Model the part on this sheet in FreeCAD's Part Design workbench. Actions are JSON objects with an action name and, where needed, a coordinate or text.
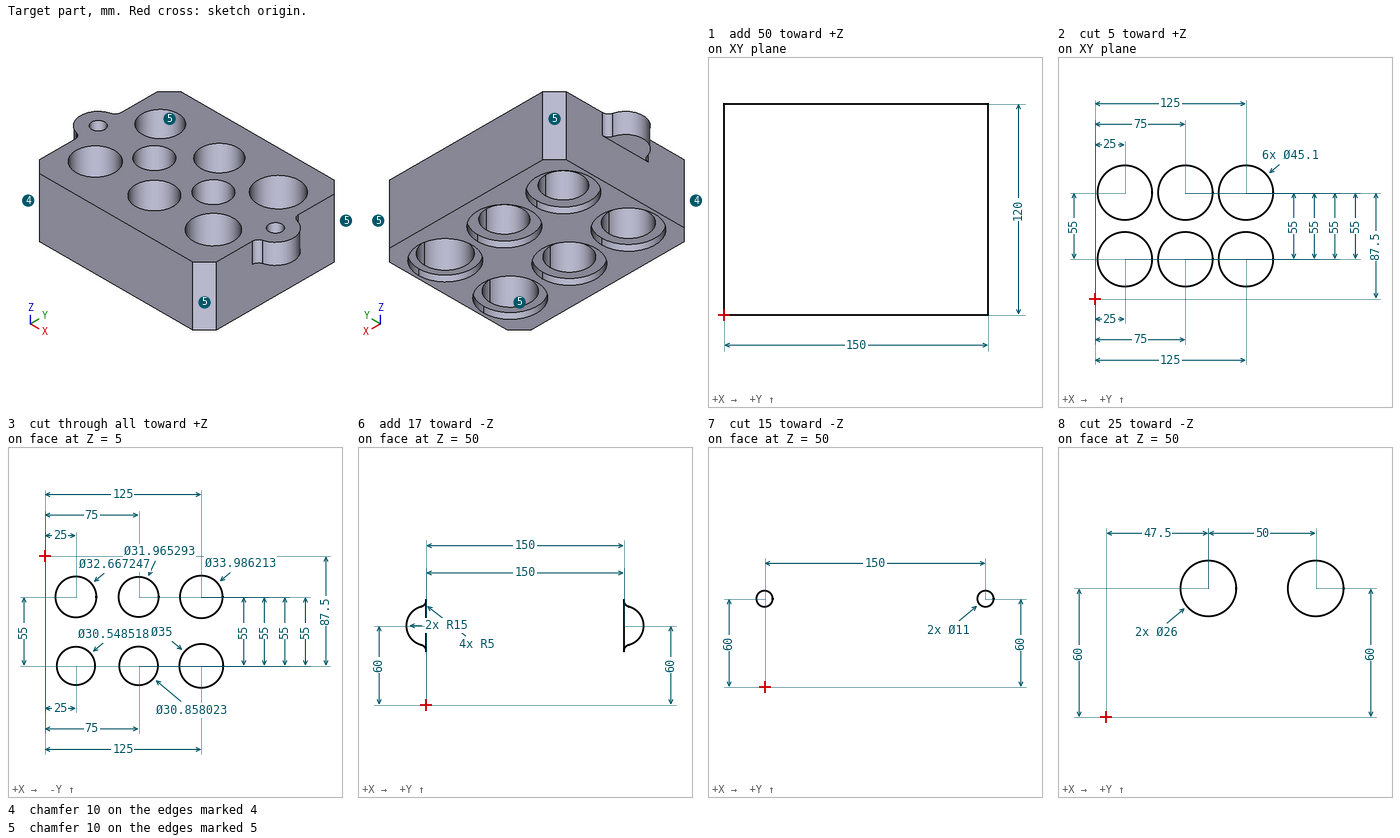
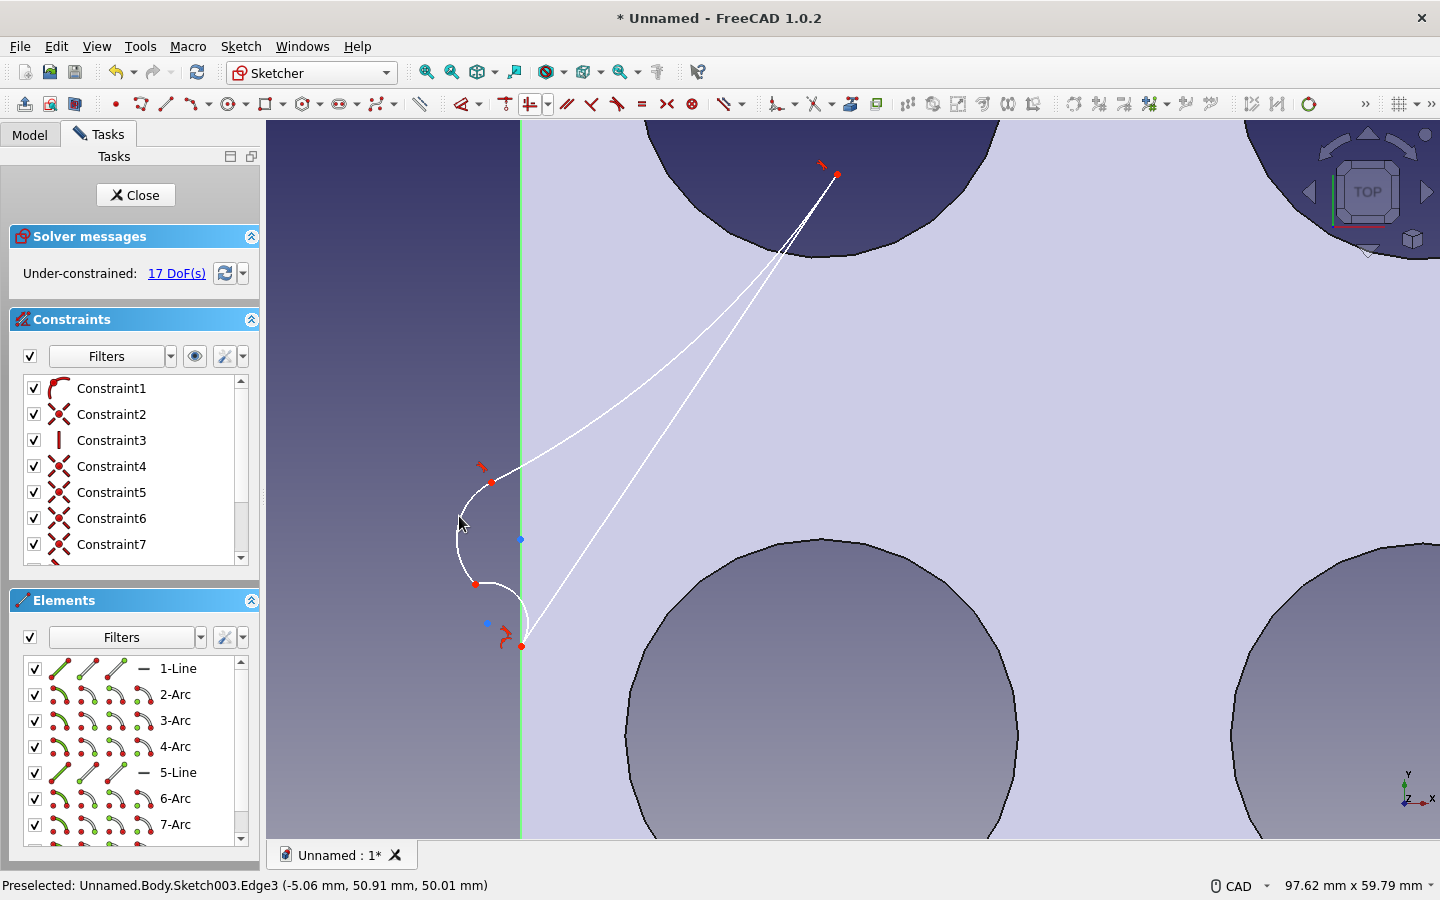
{"action": "left_click", "coordinate": [465, 507]}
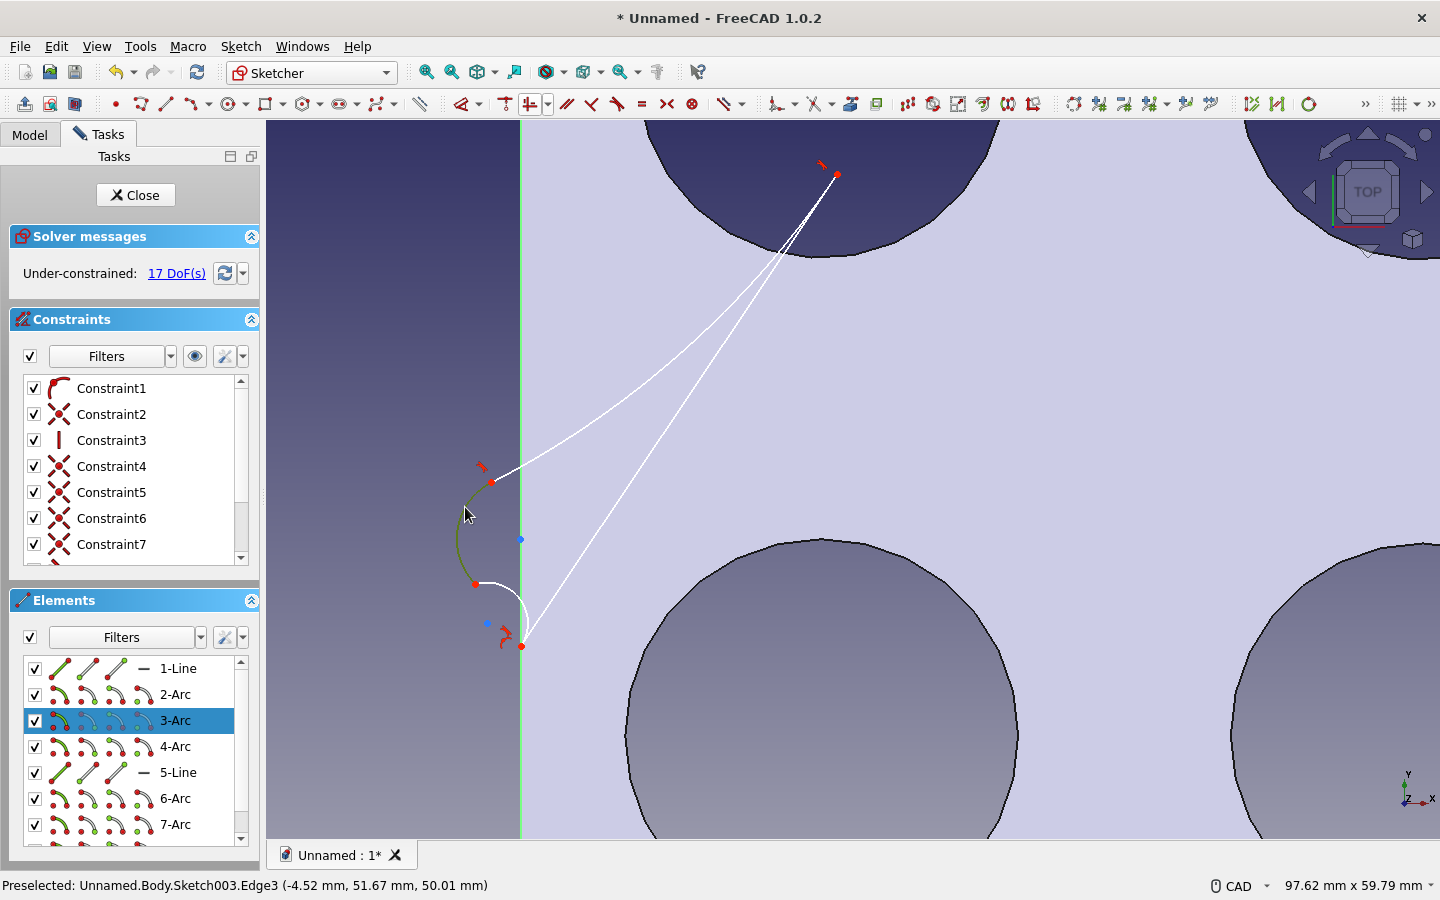
{"action": "left_click", "coordinate": [505, 587]}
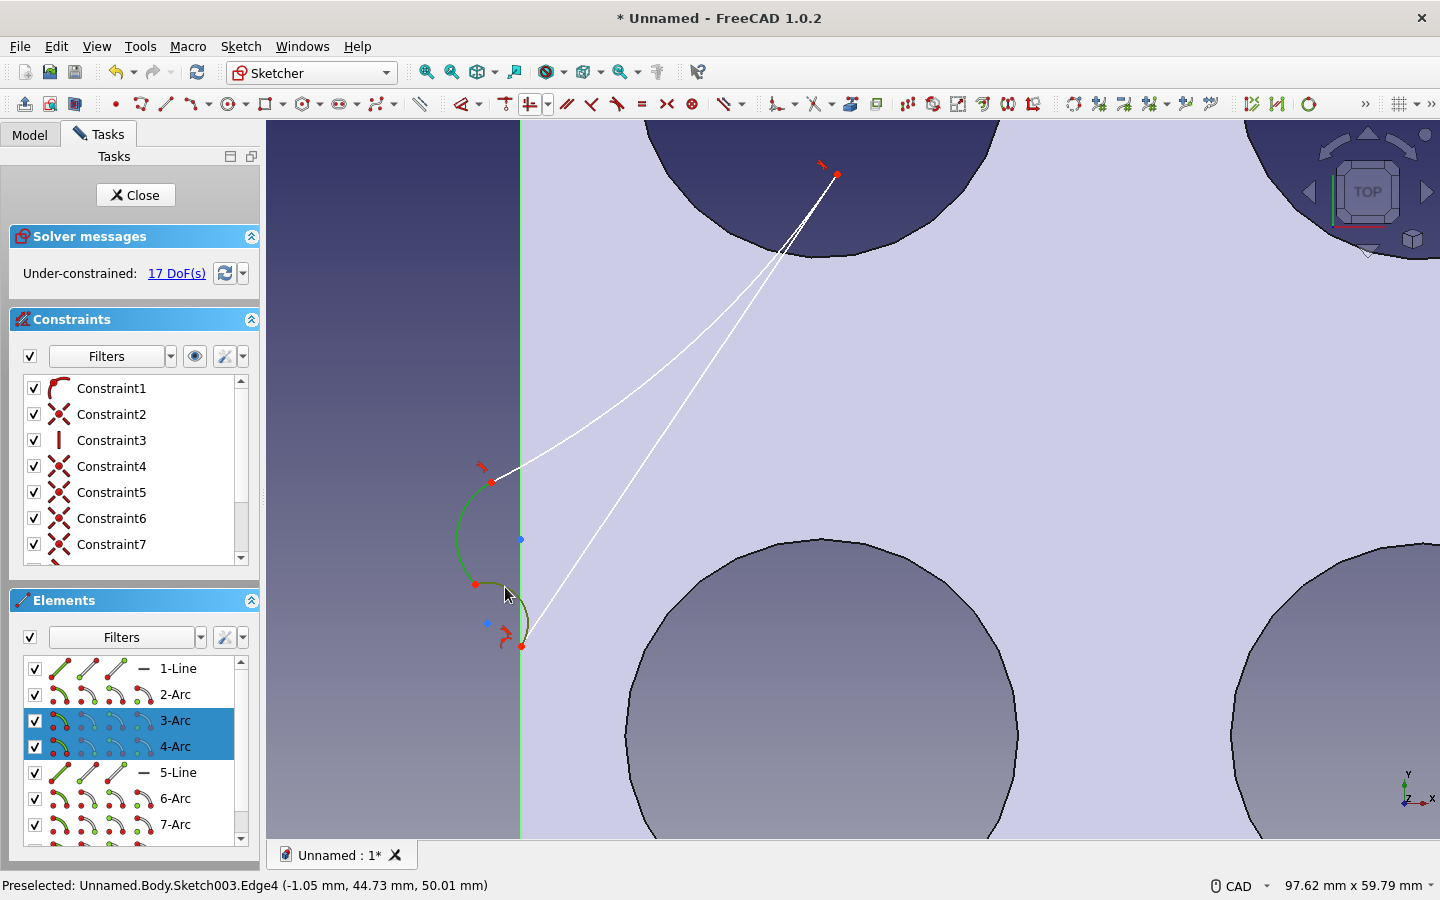
{"action": "left_click", "coordinate": [617, 104]}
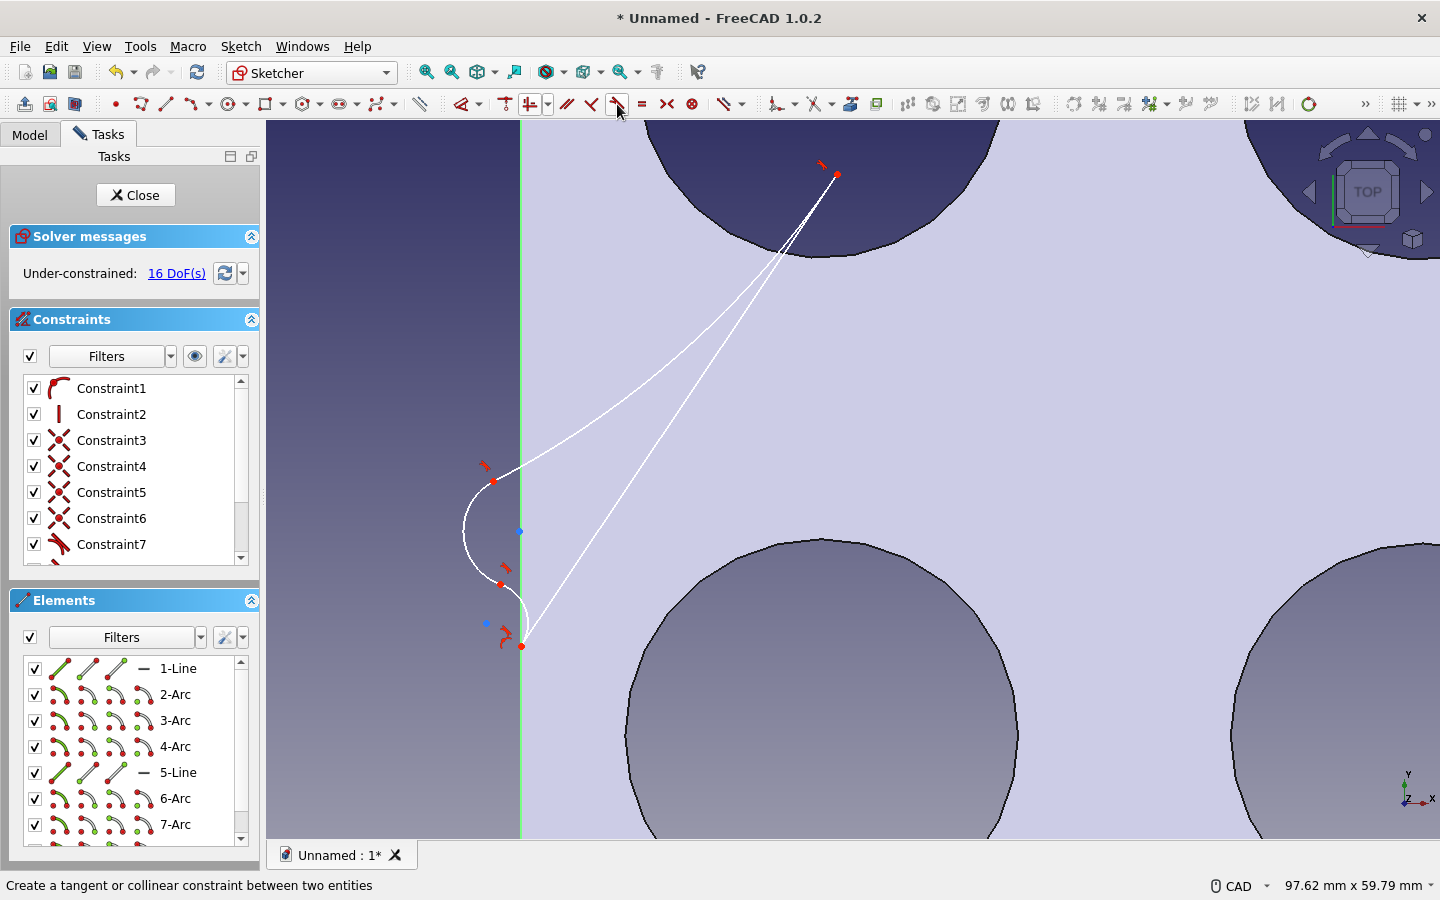
{"action": "scroll", "coordinate": [509, 406], "scroll_direction": "down", "scroll_amount": 6}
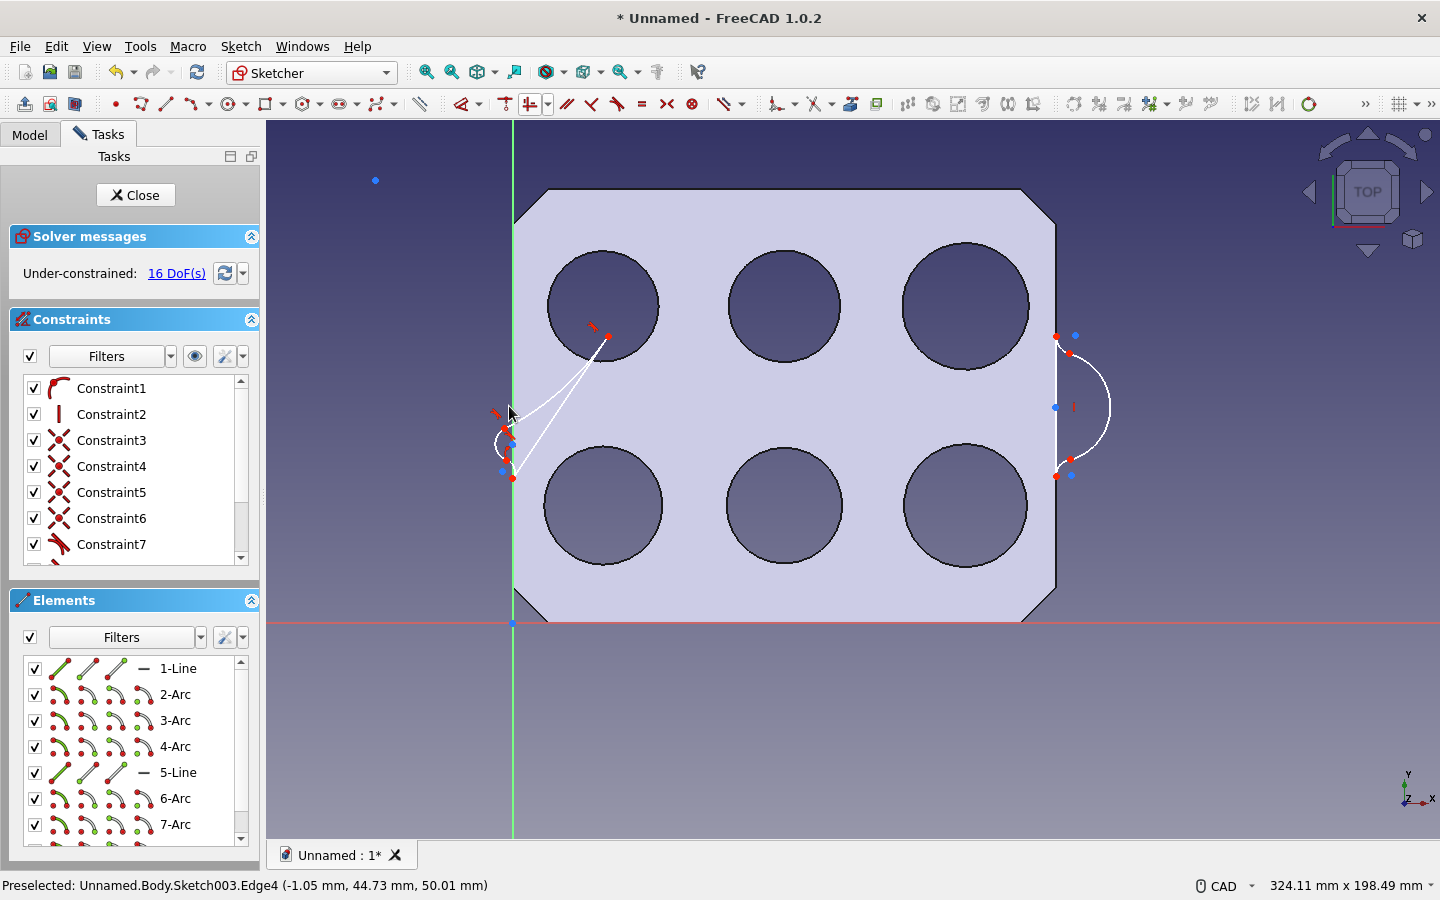
{"action": "left_click", "coordinate": [1056, 379]}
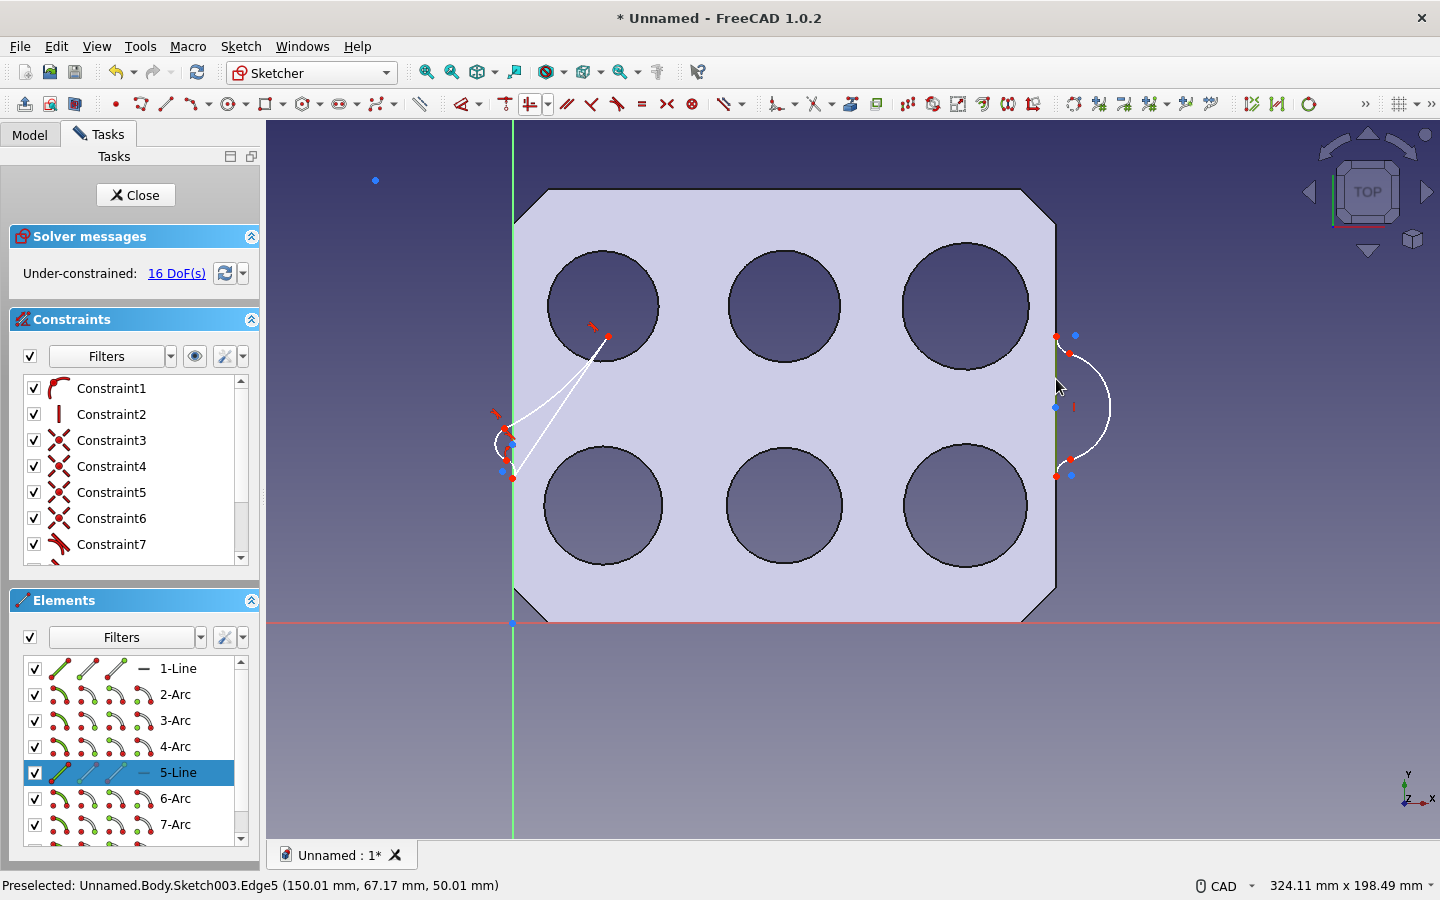
{"action": "scroll", "coordinate": [1063, 462], "scroll_direction": "up", "scroll_amount": 4}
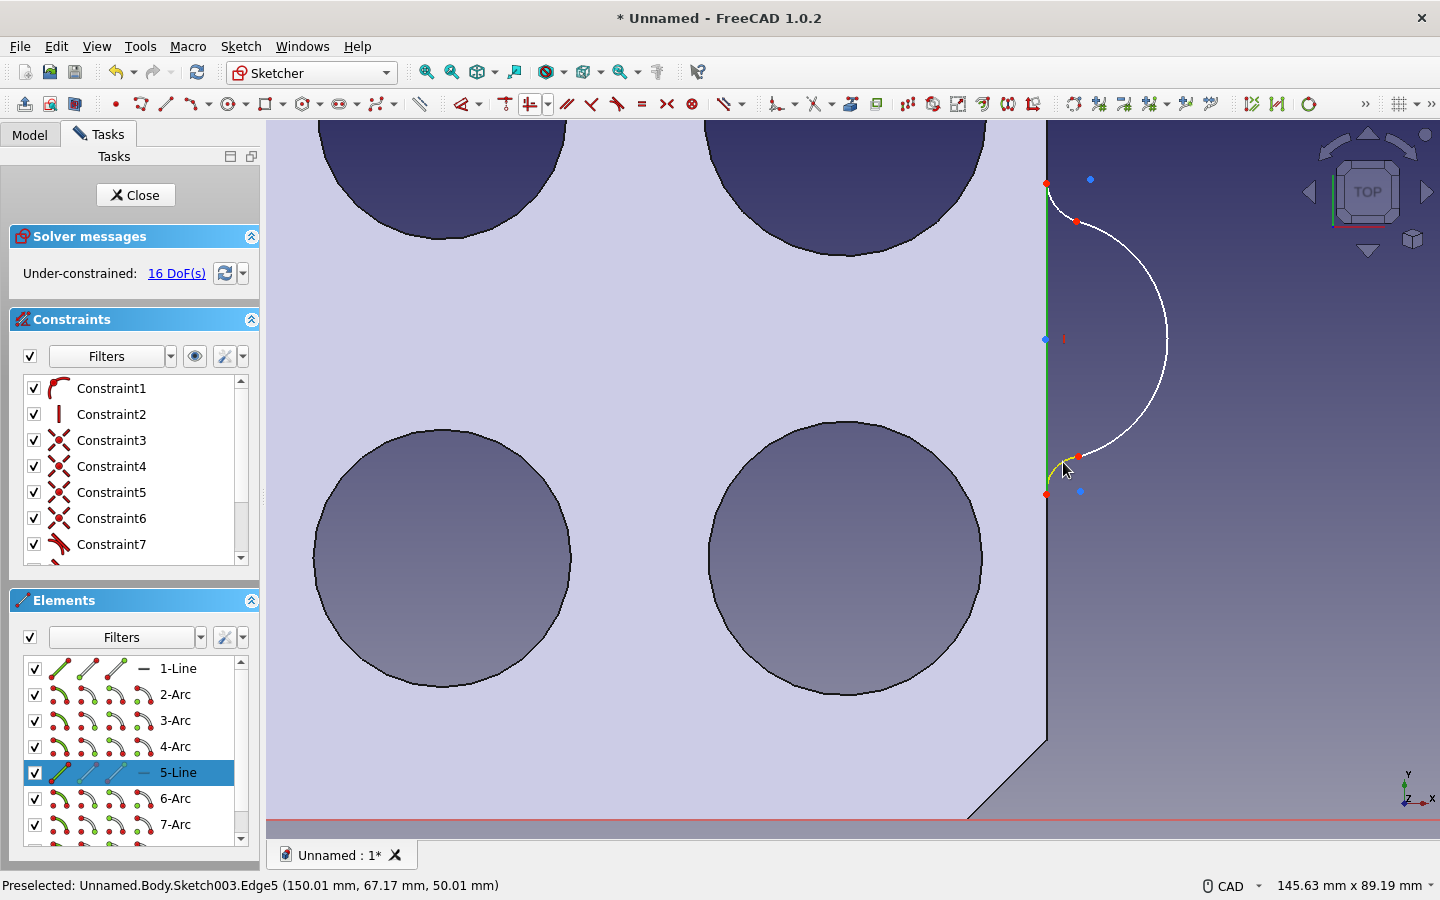
{"action": "left_click", "coordinate": [1063, 462]}